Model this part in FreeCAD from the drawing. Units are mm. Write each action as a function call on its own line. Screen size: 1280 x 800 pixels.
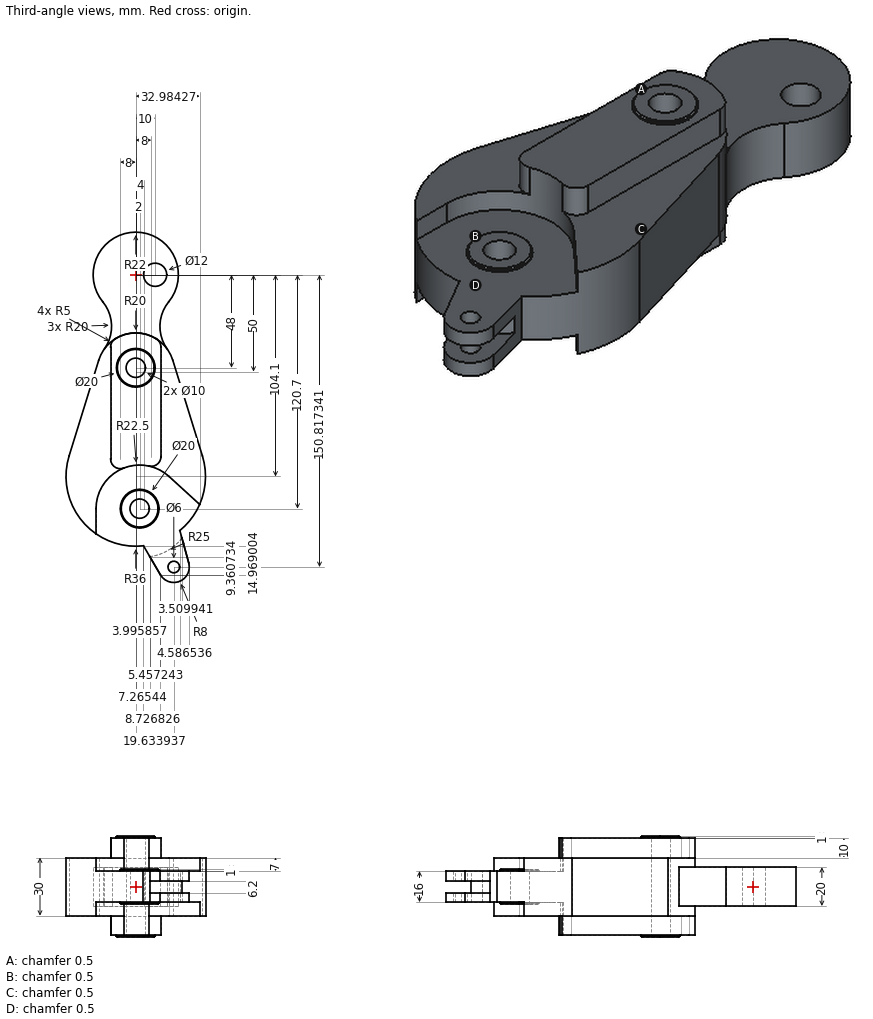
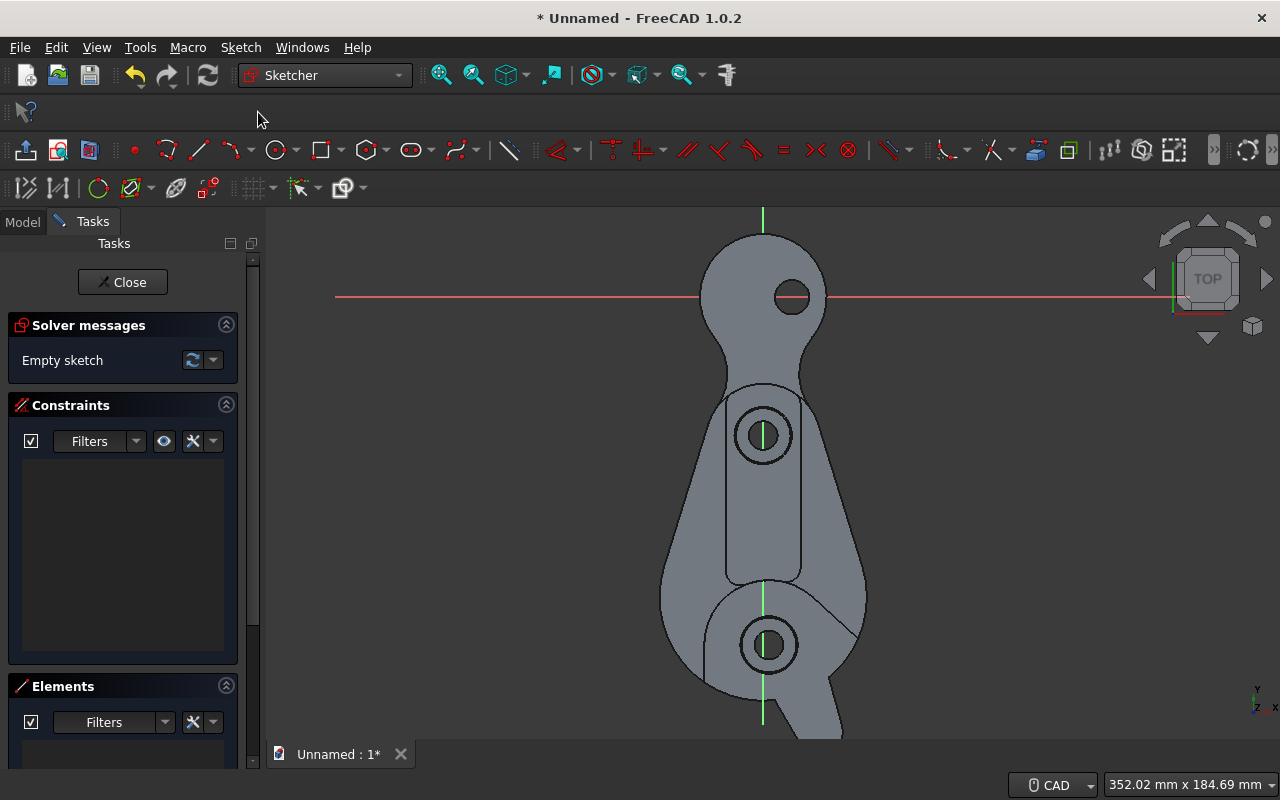
scroll(704, 473, down, 5)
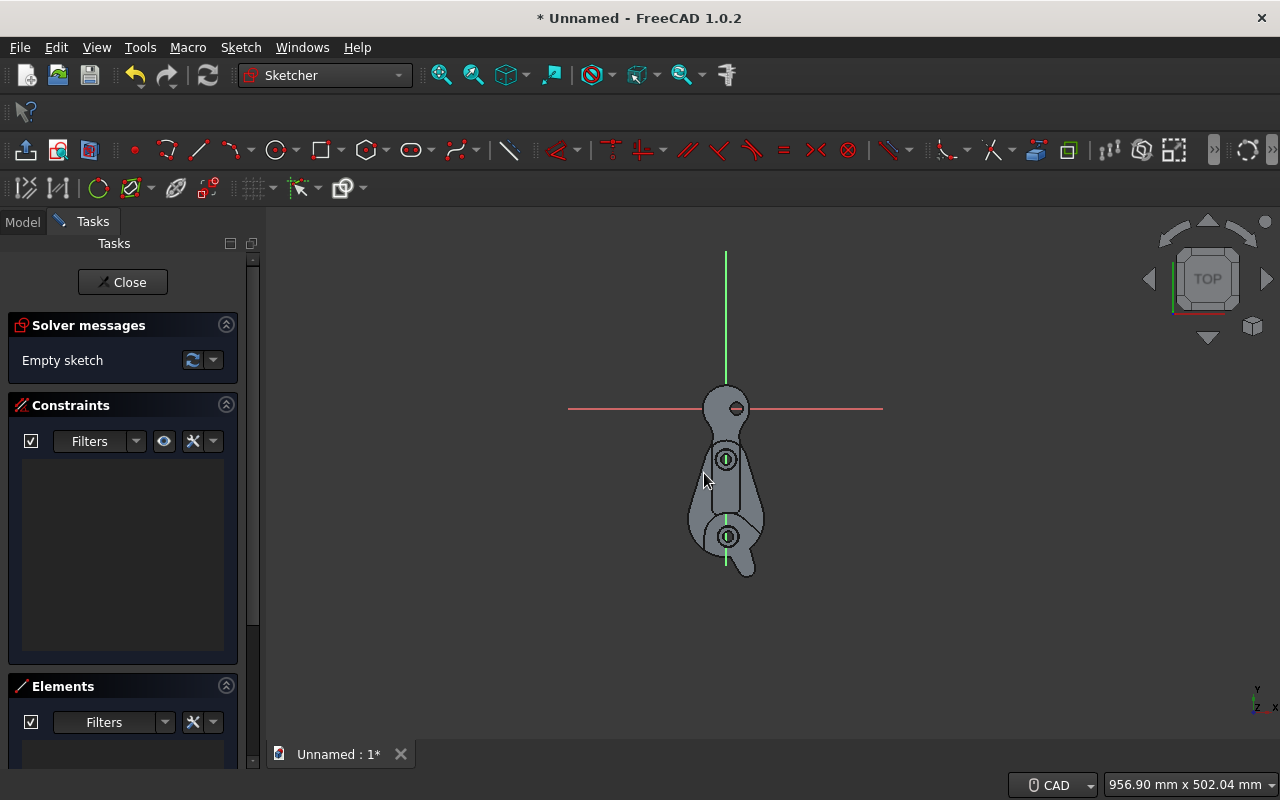
scroll(749, 573, up, 15)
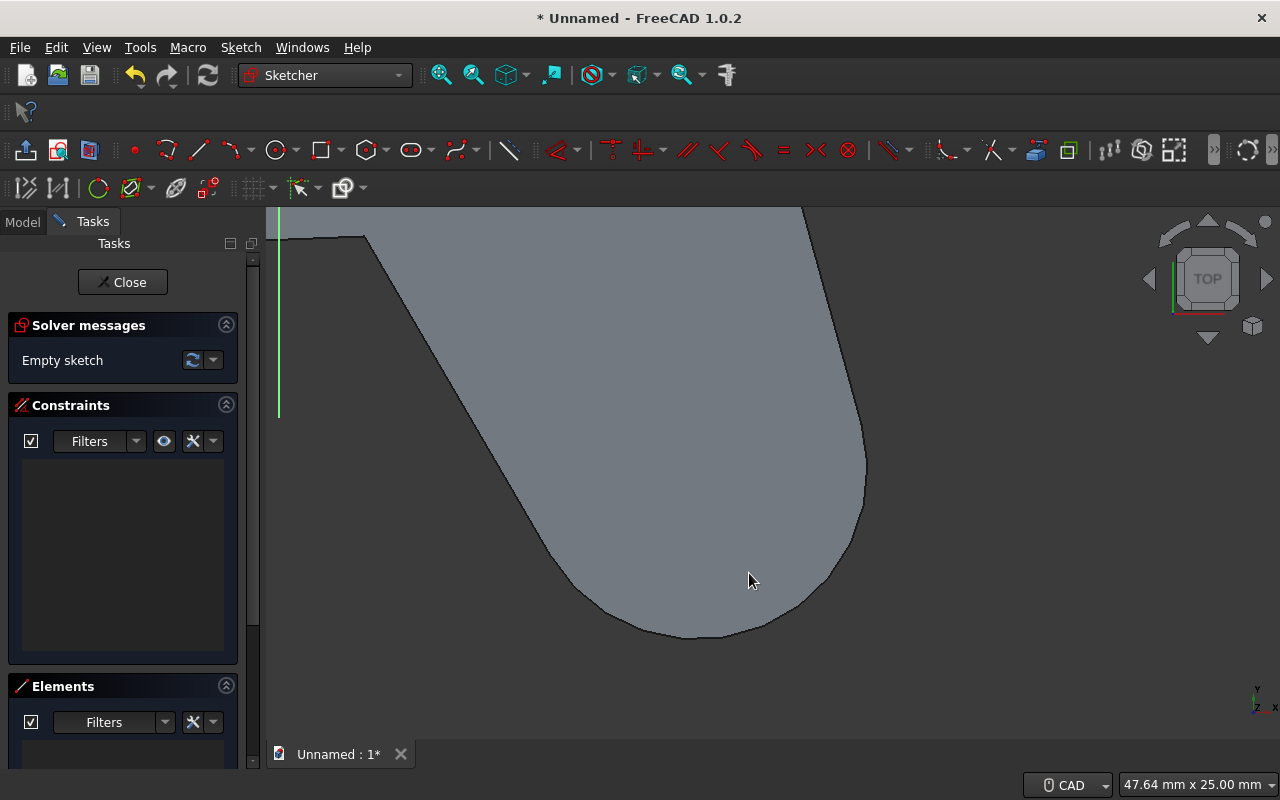
scroll(693, 467, up, 5)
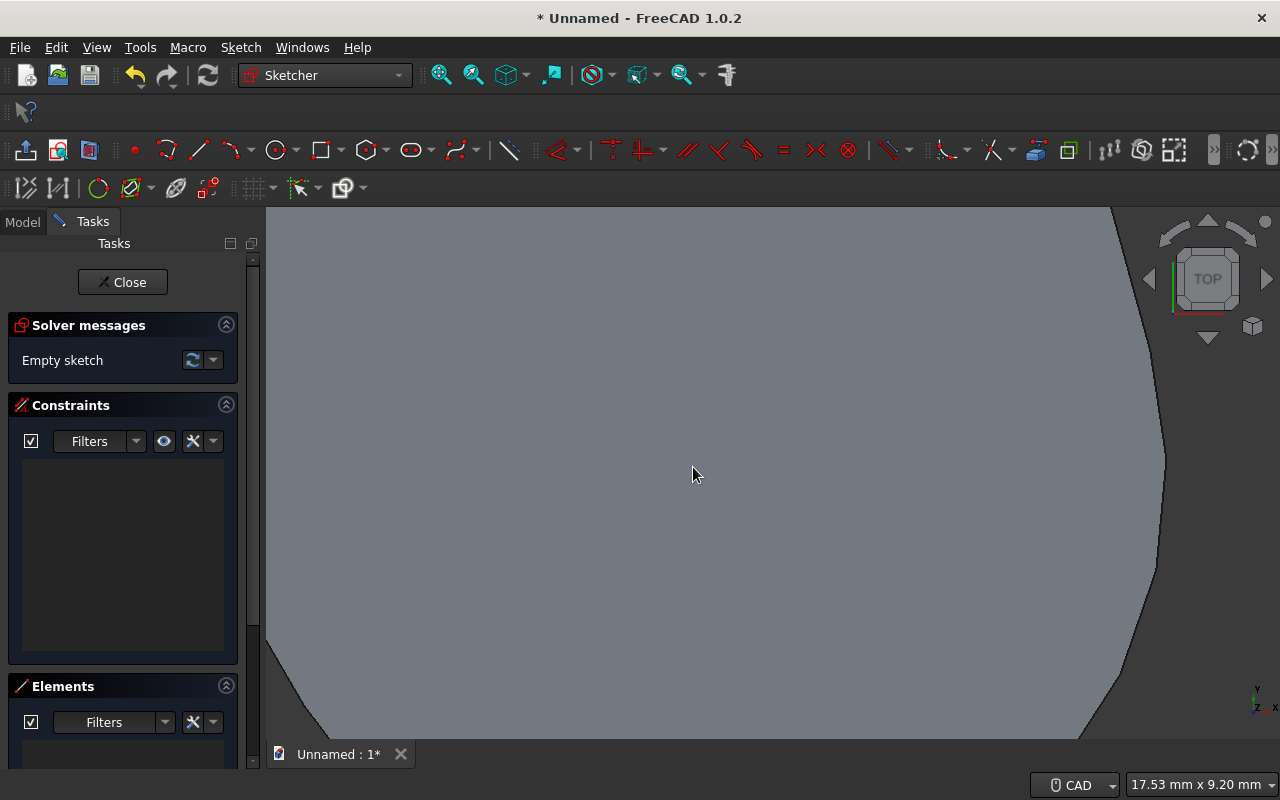
click(276, 150)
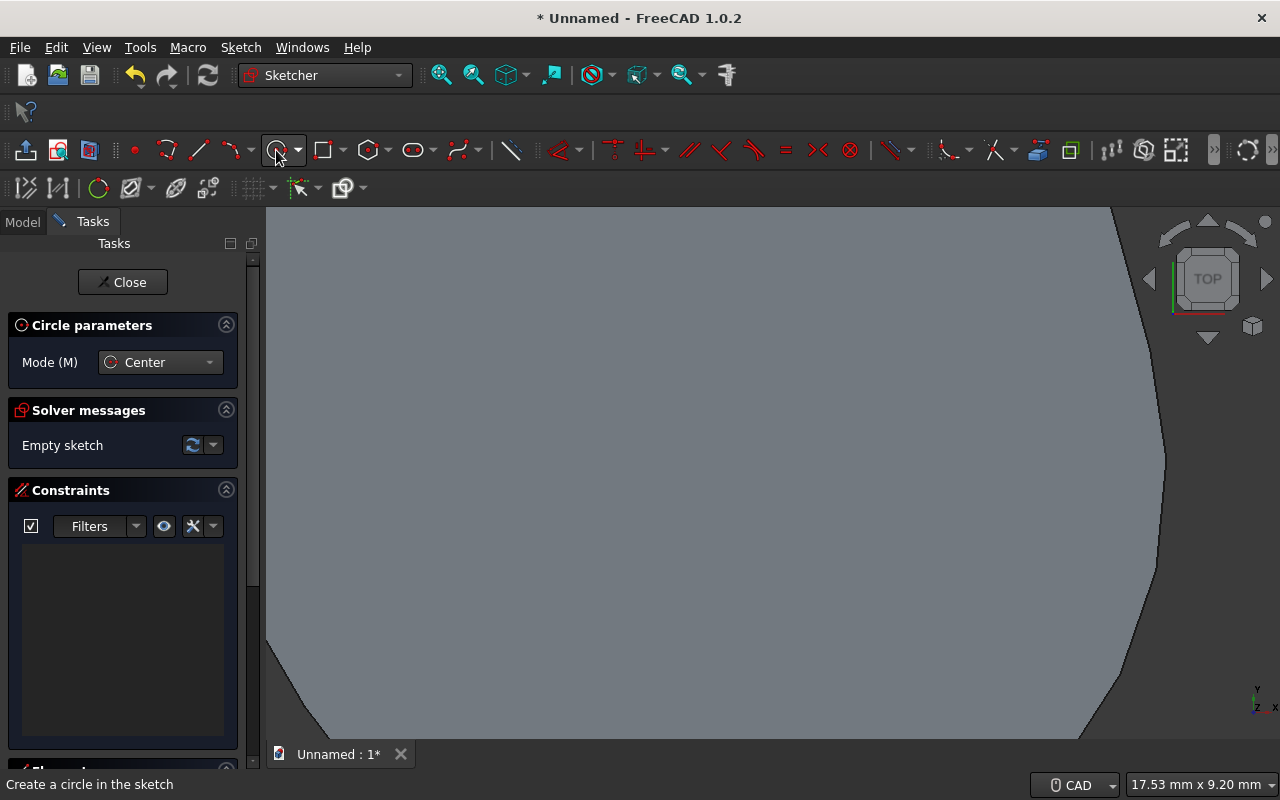
click(704, 472)
click(827, 350)
key(Escape)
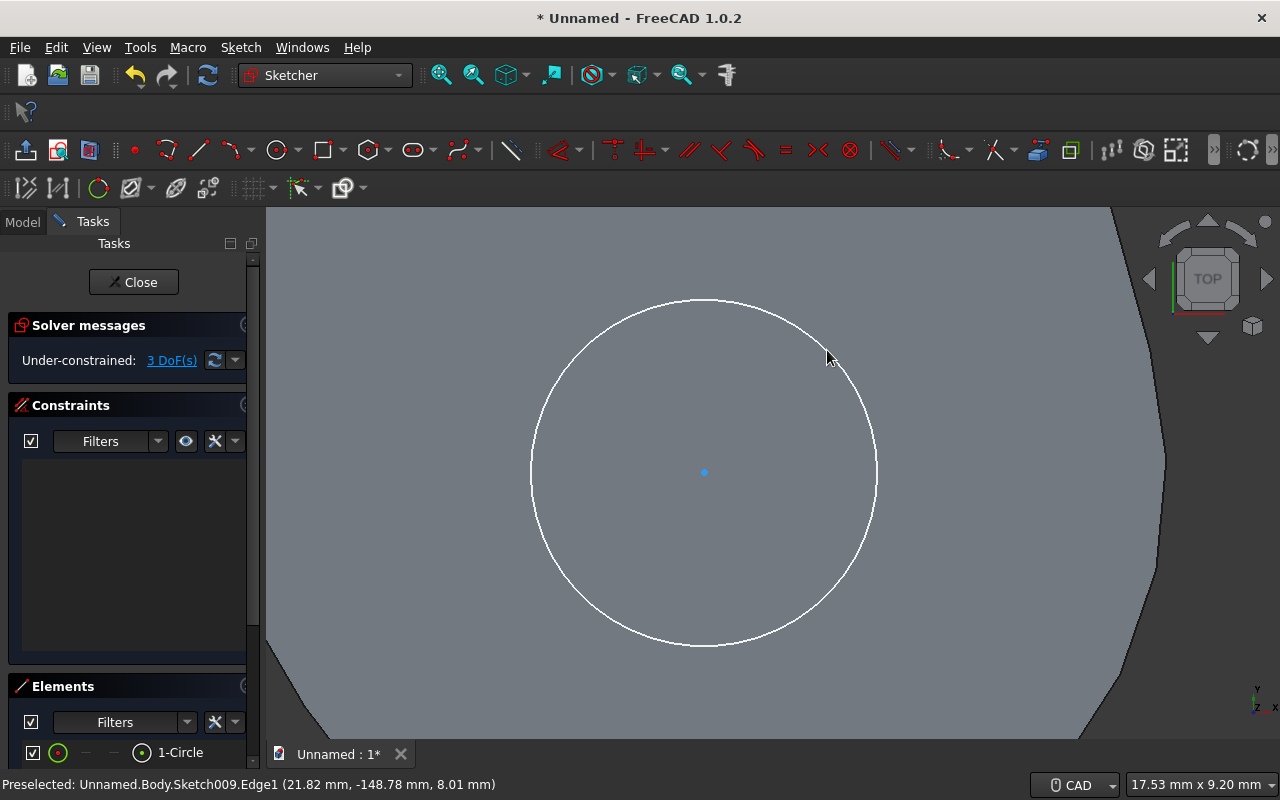
click(558, 150)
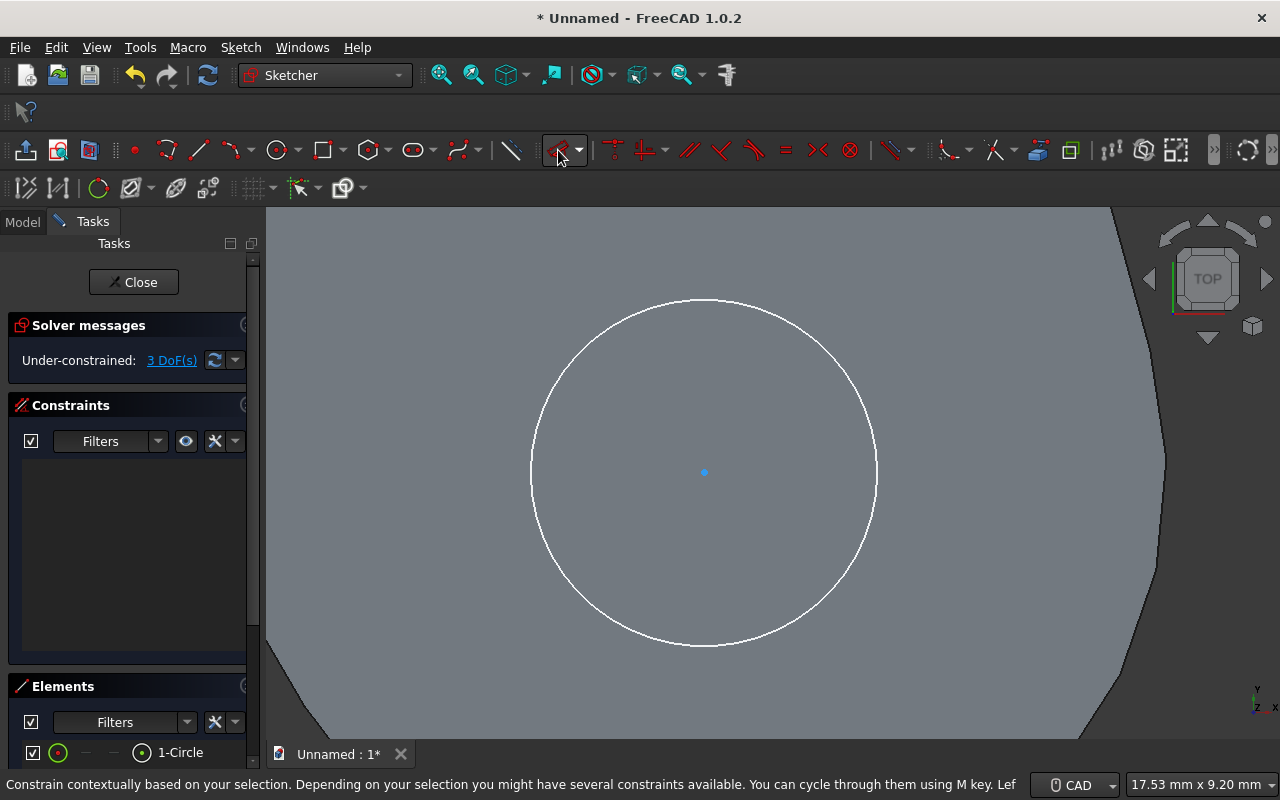
click(826, 350)
click(849, 327)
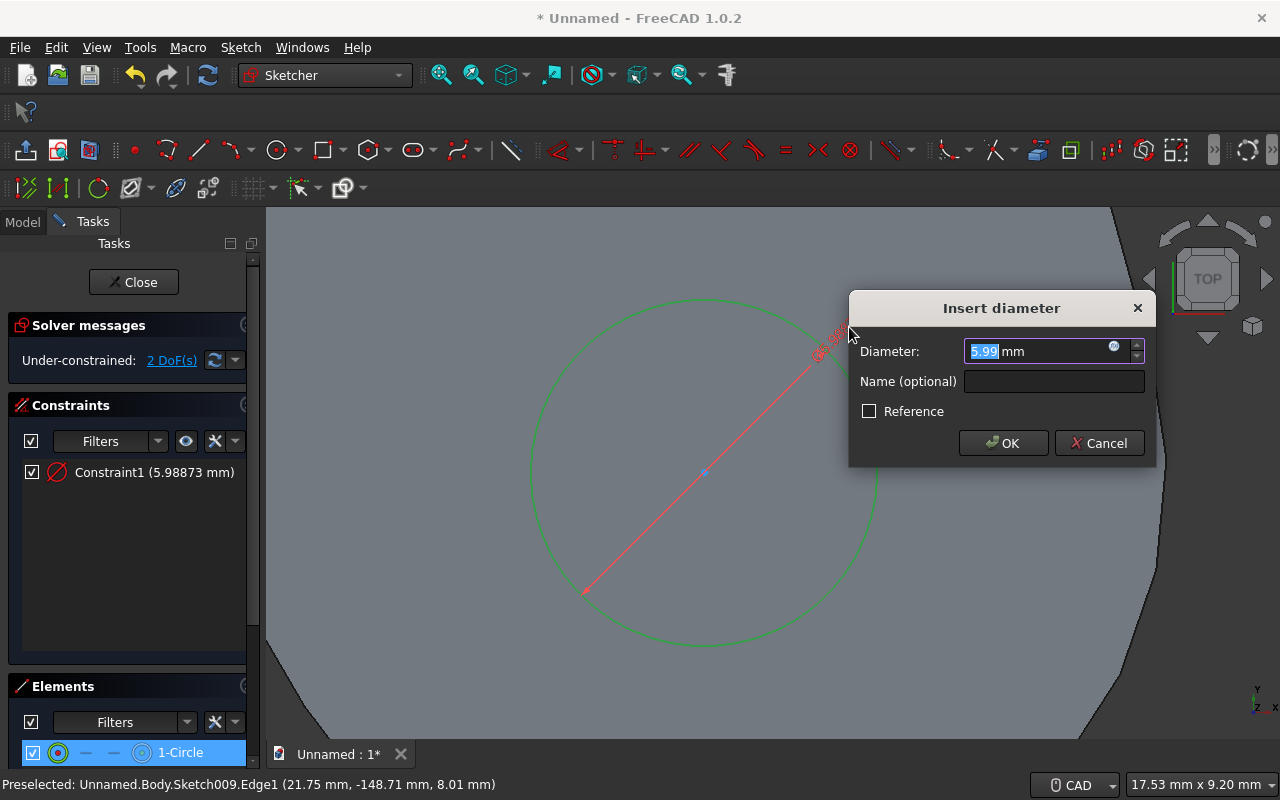
text(6)
key(Return)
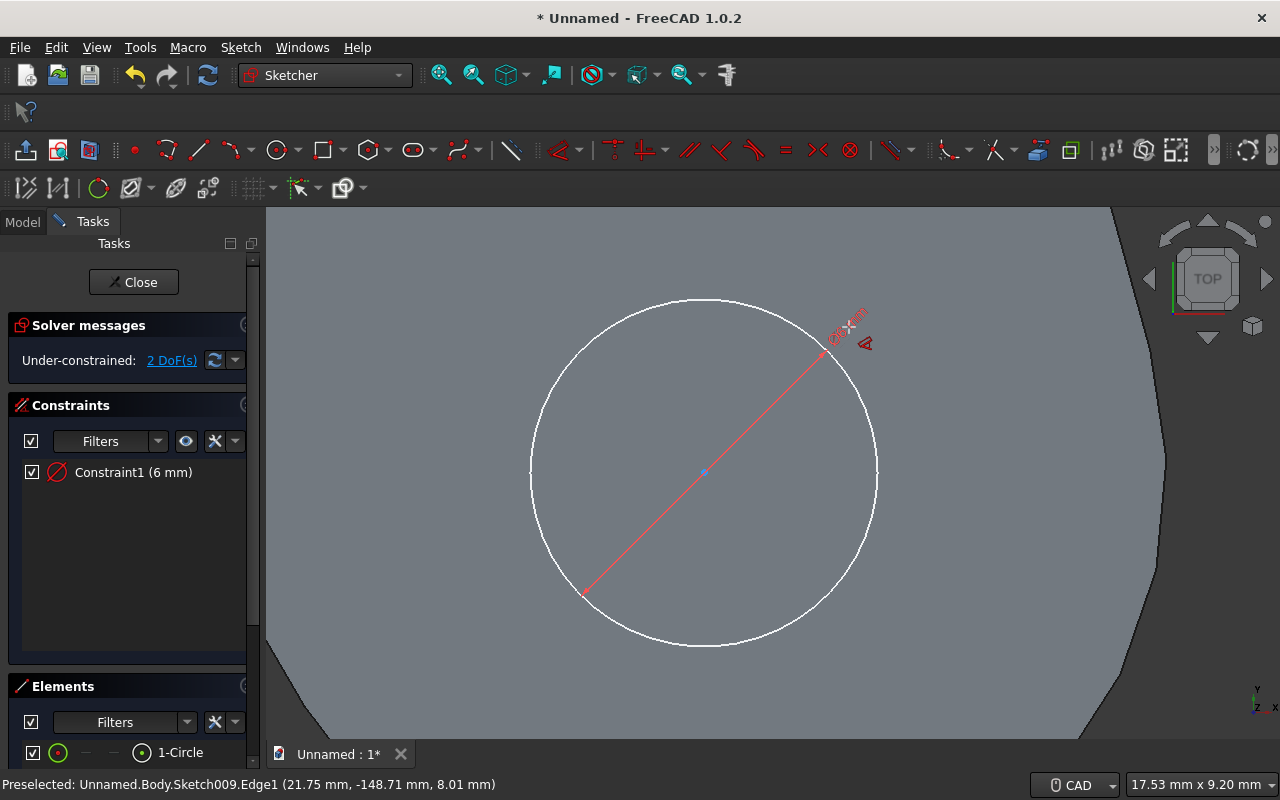
click(704, 473)
click(499, 507)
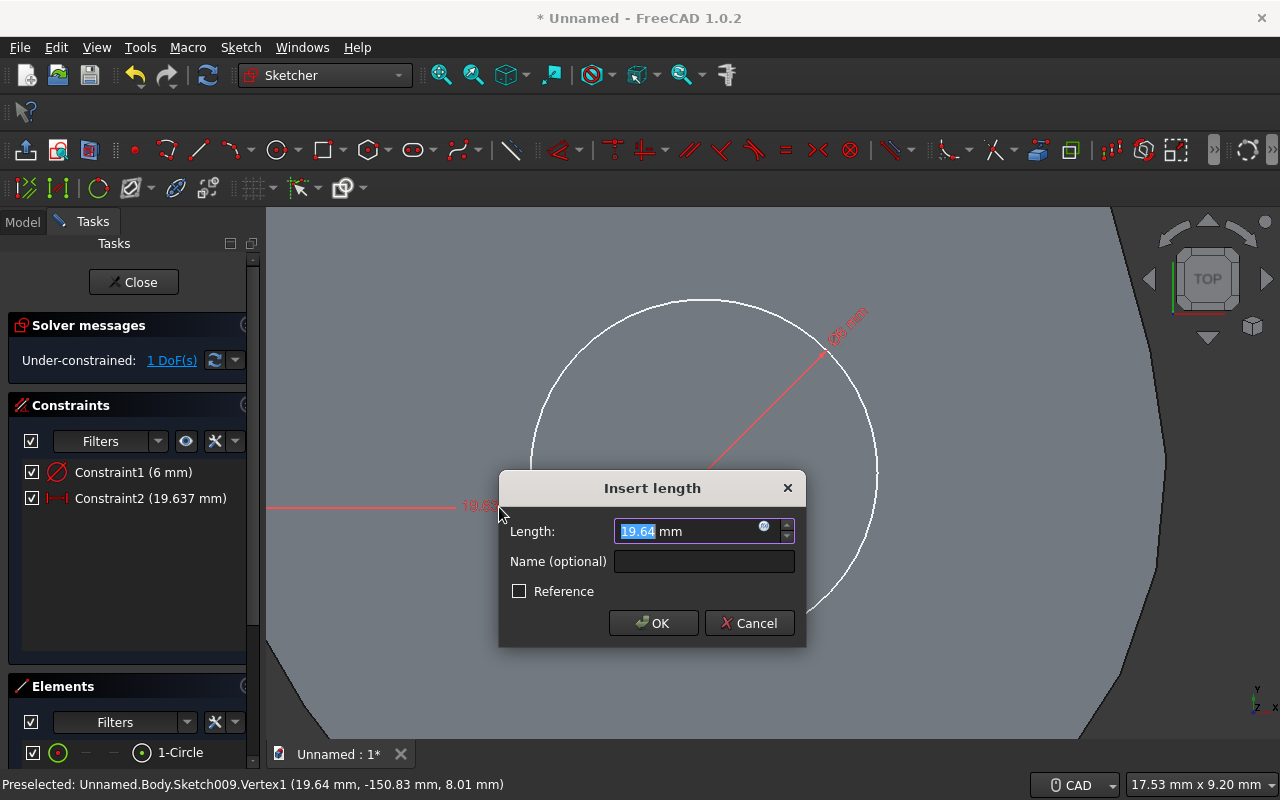
text(19.633937)
key(Return)